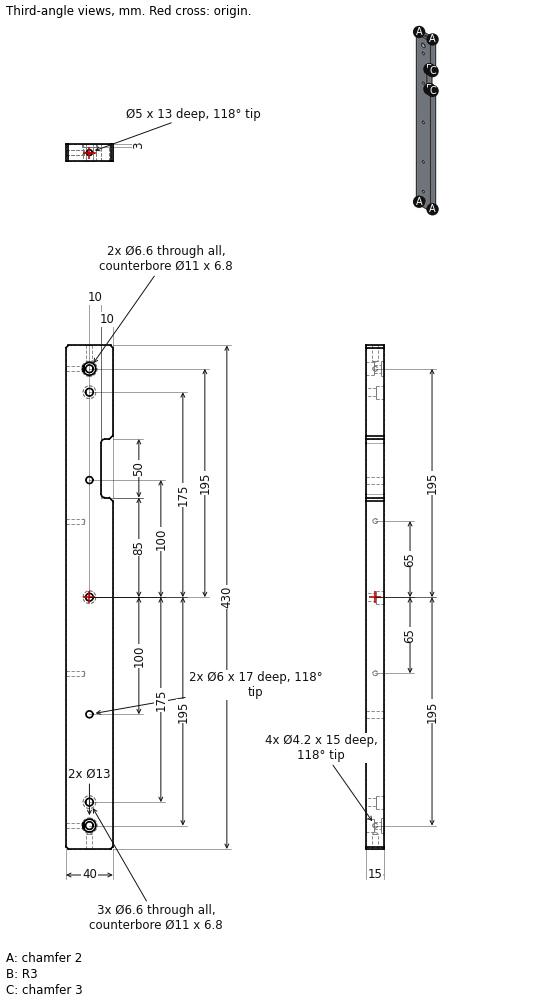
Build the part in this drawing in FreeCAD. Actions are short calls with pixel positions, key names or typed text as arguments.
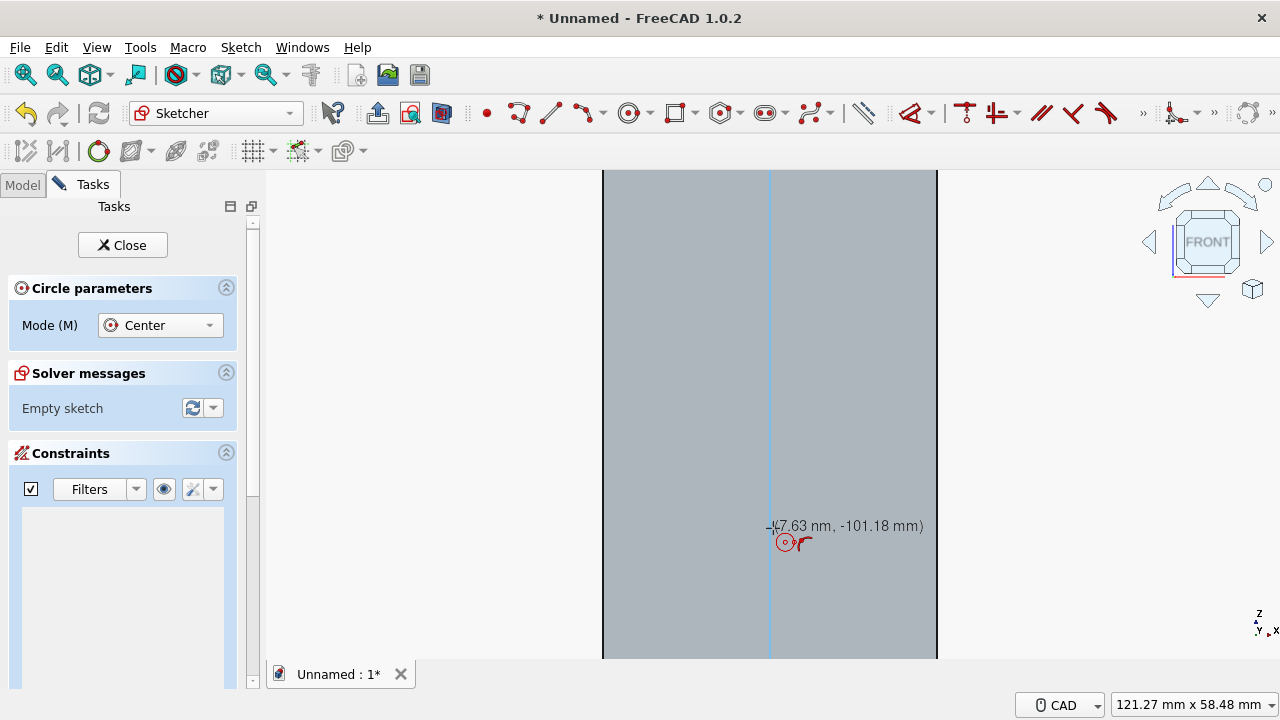
scroll(692, 559, down, 9)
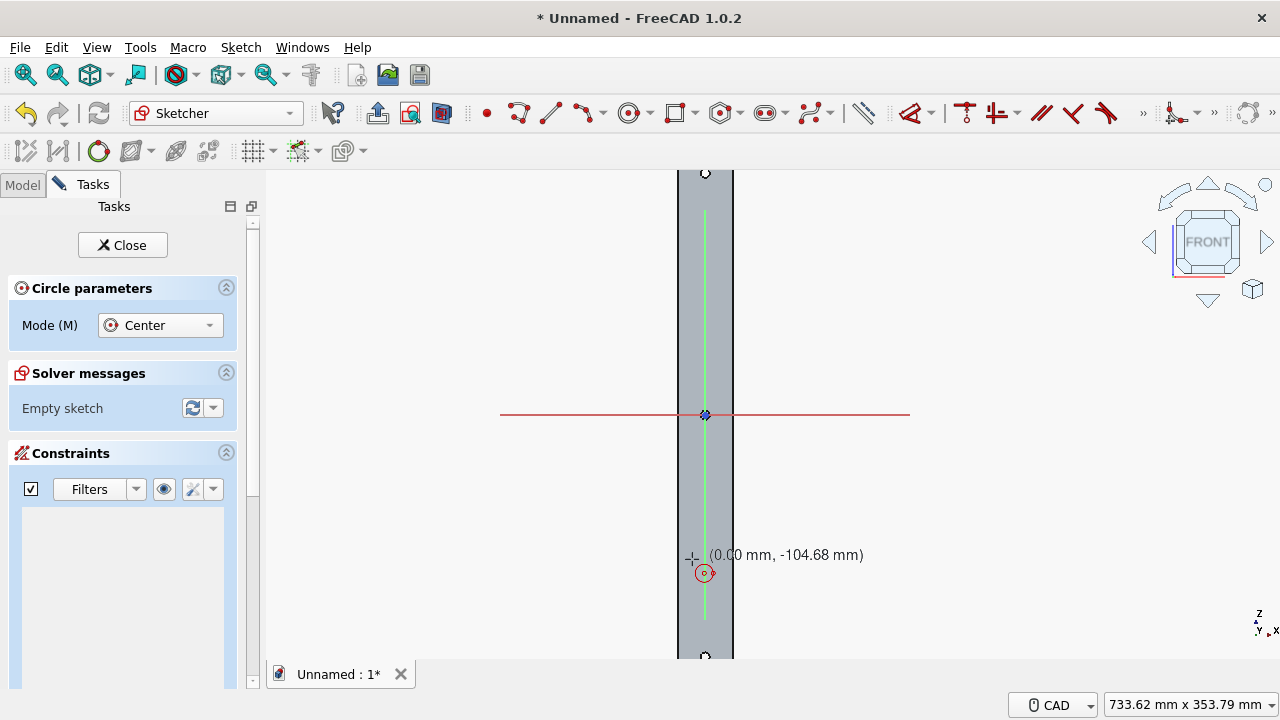
click(705, 553)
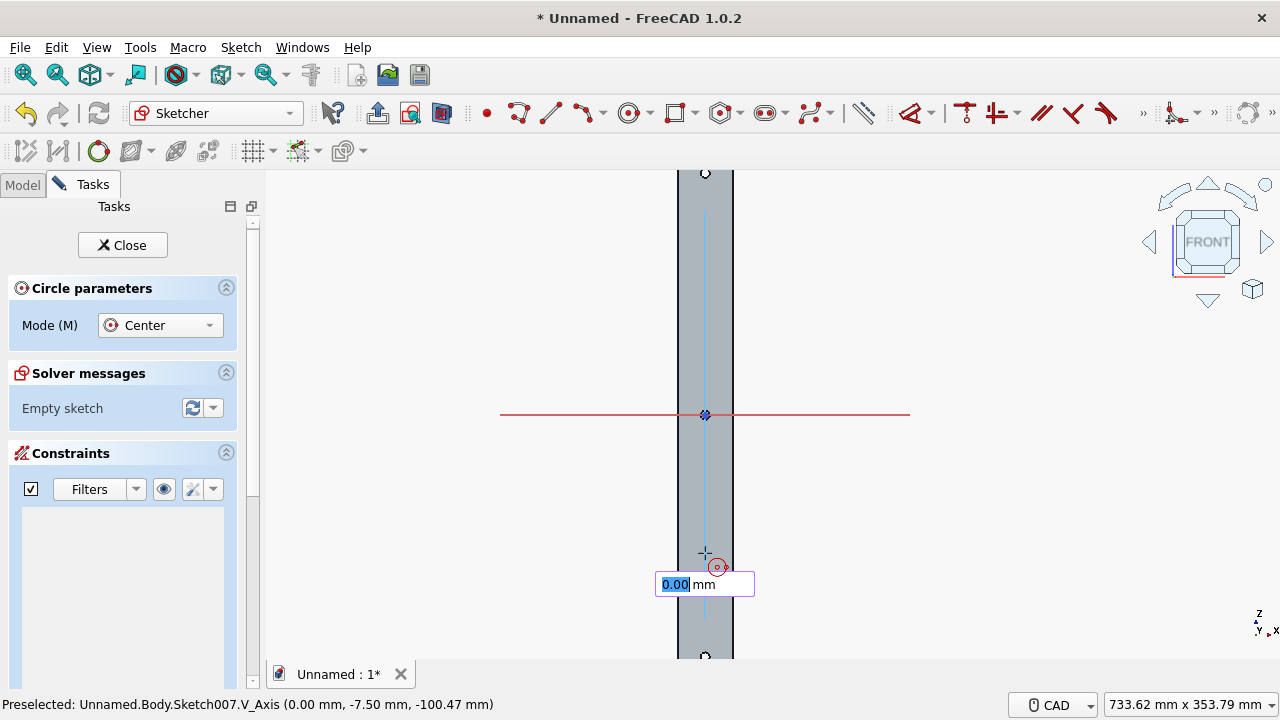
scroll(709, 552, up, 8)
move(708, 549)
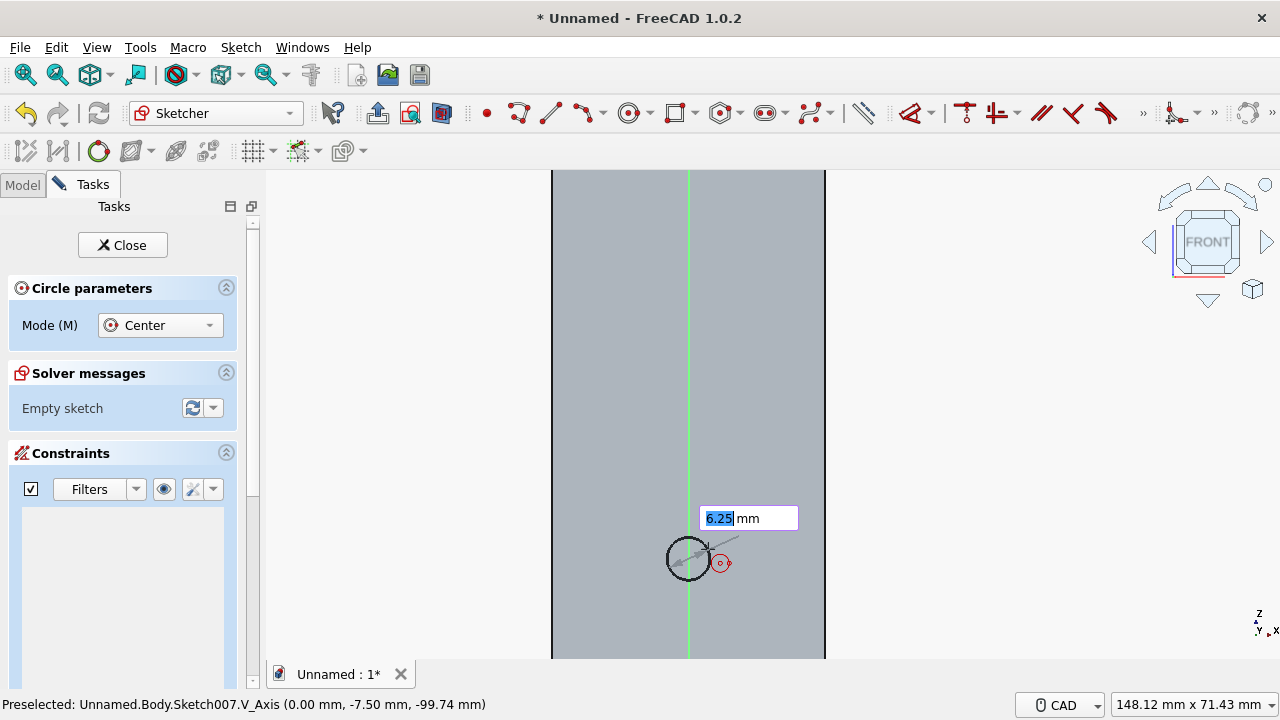
text(6)
key(Return)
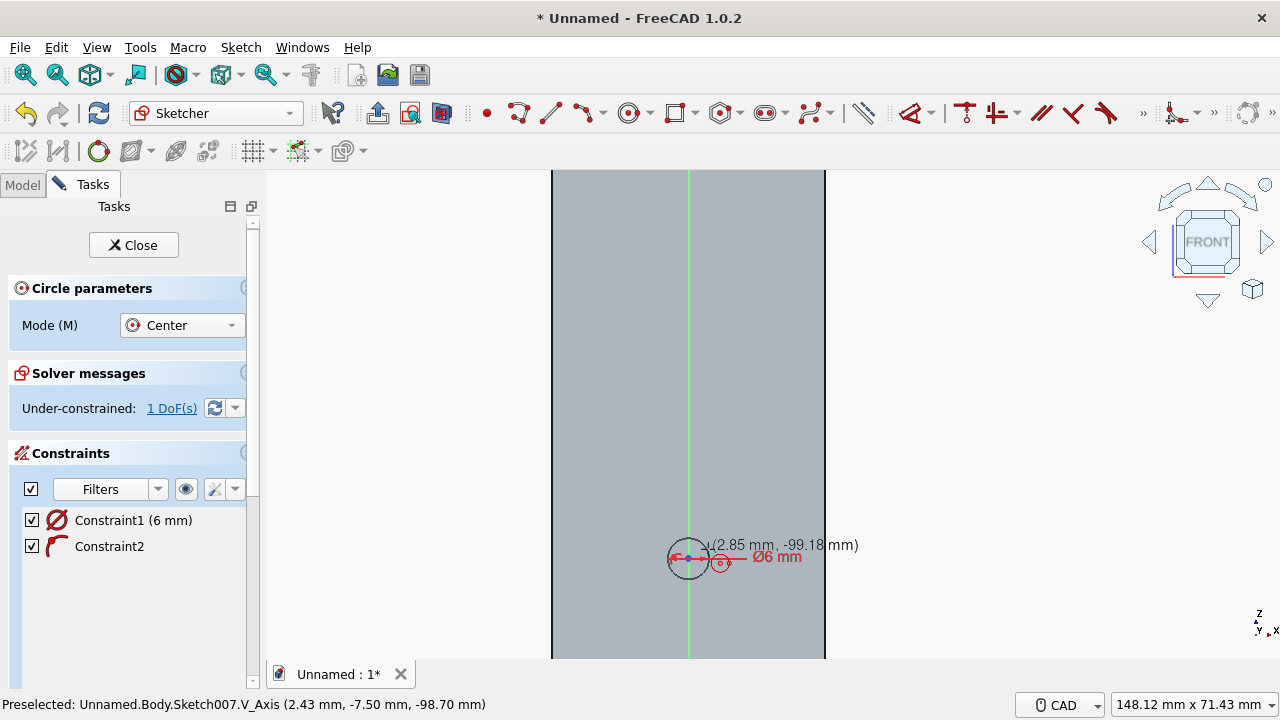
scroll(709, 552, down, 8)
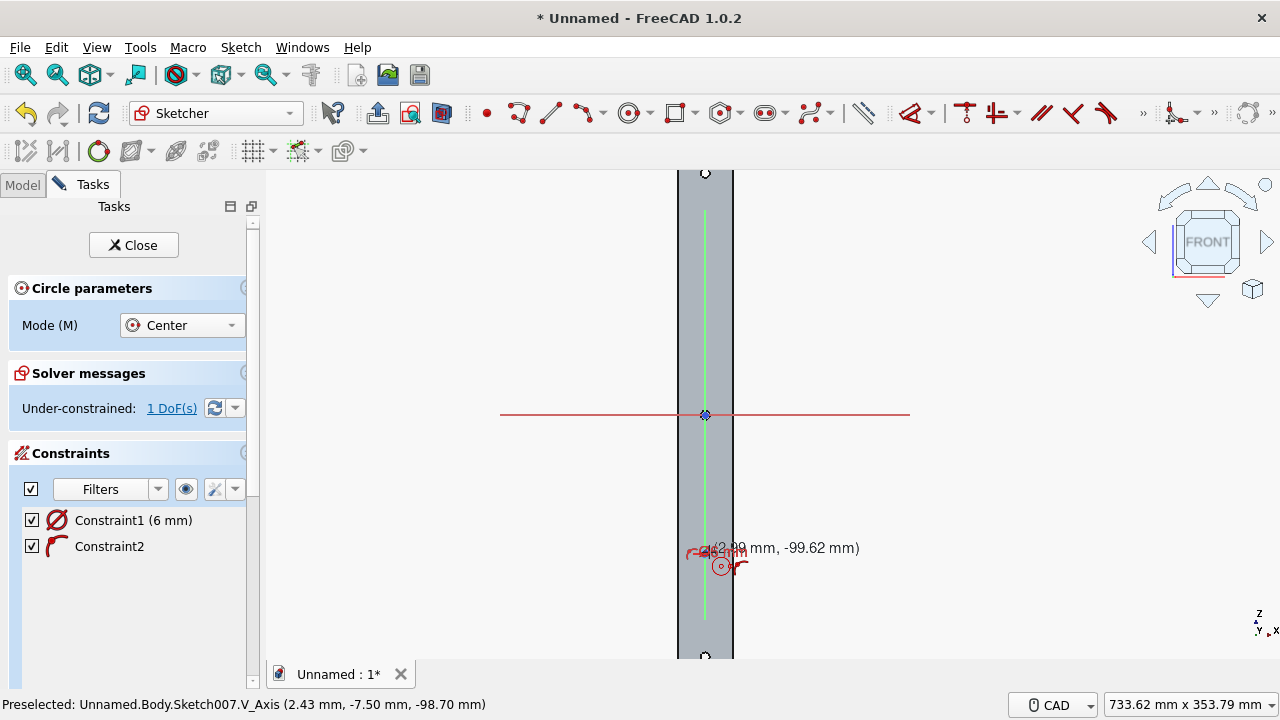
scroll(705, 277, up, 9)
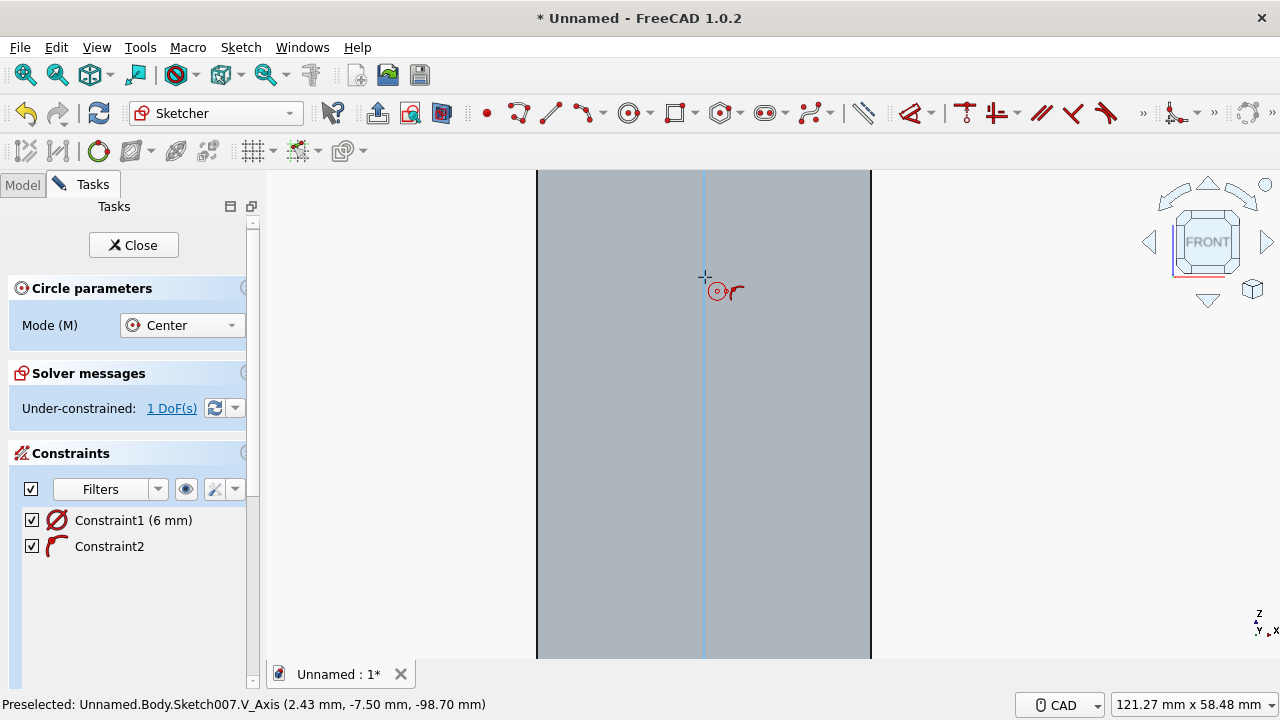
scroll(705, 276, down, 9)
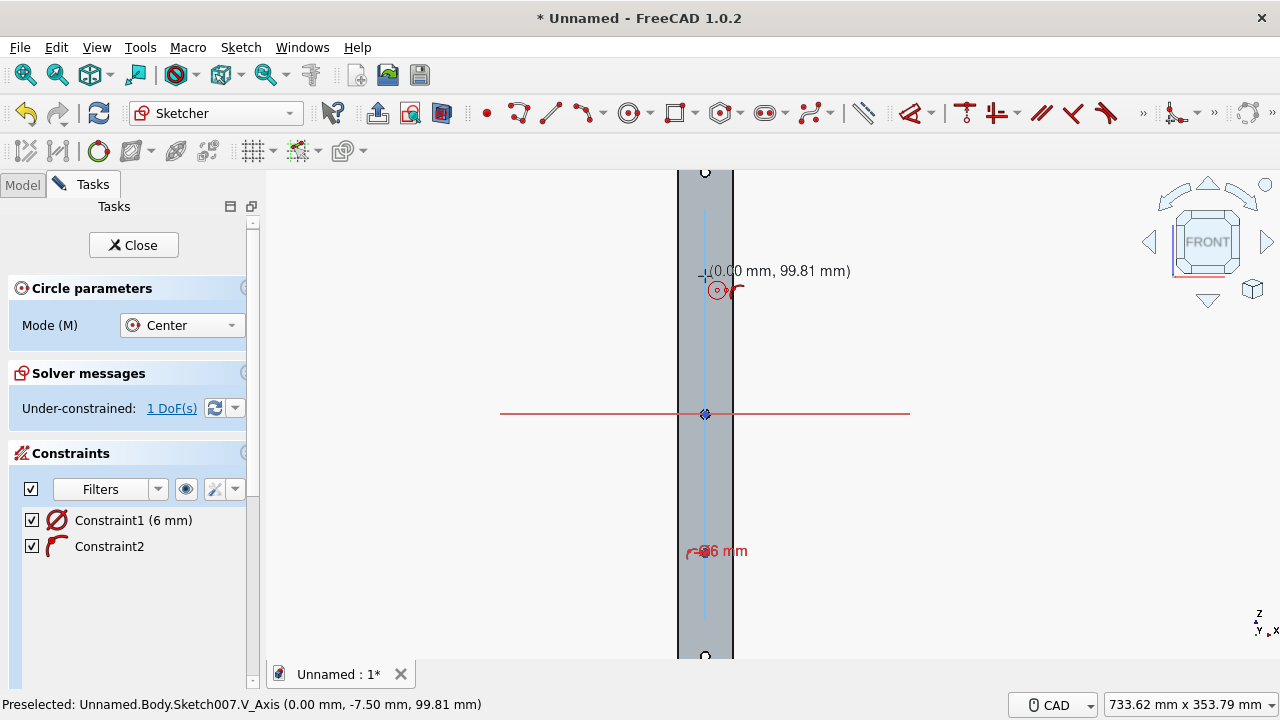
click(705, 276)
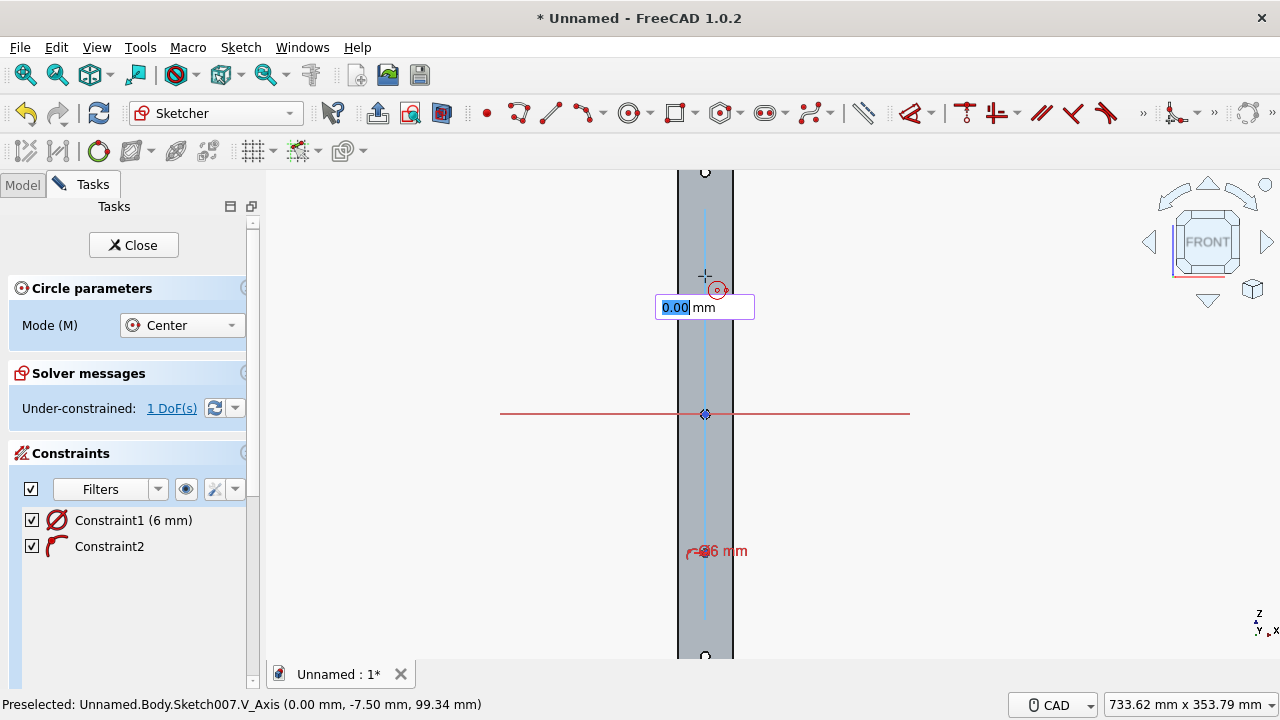
scroll(709, 275, up, 8)
move(708, 272)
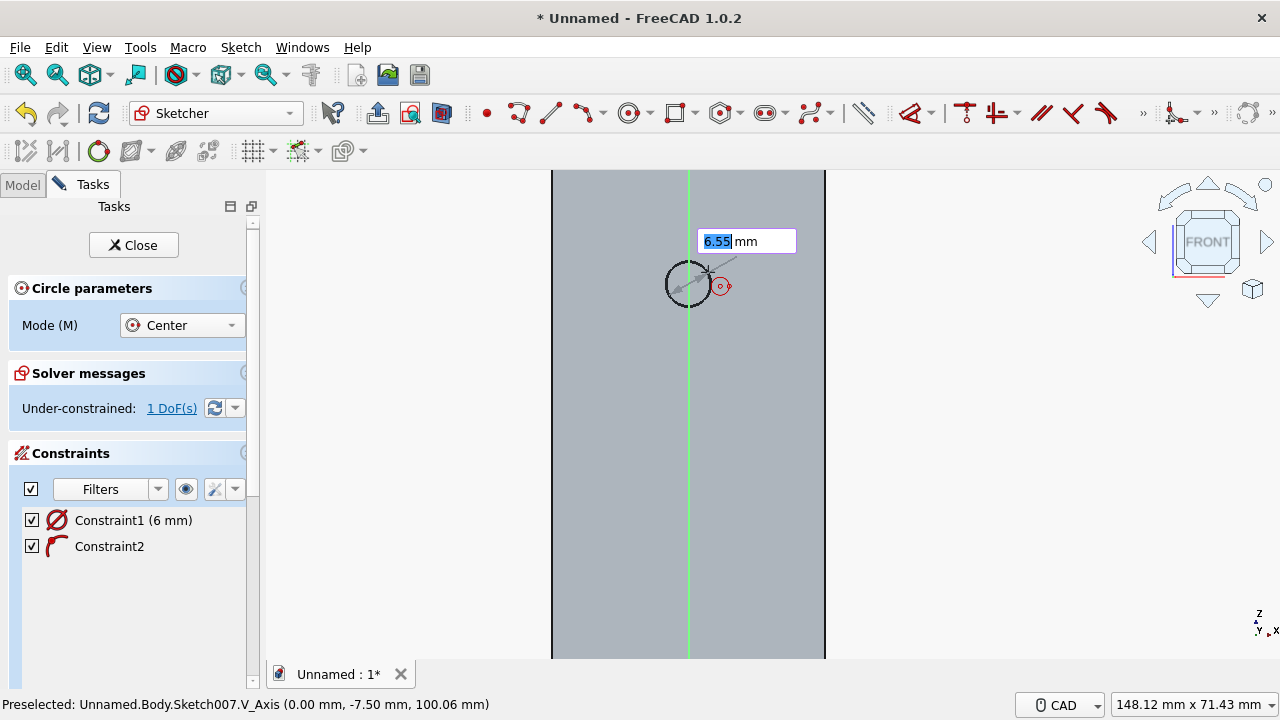
text(6)
key(Return)
key(Escape)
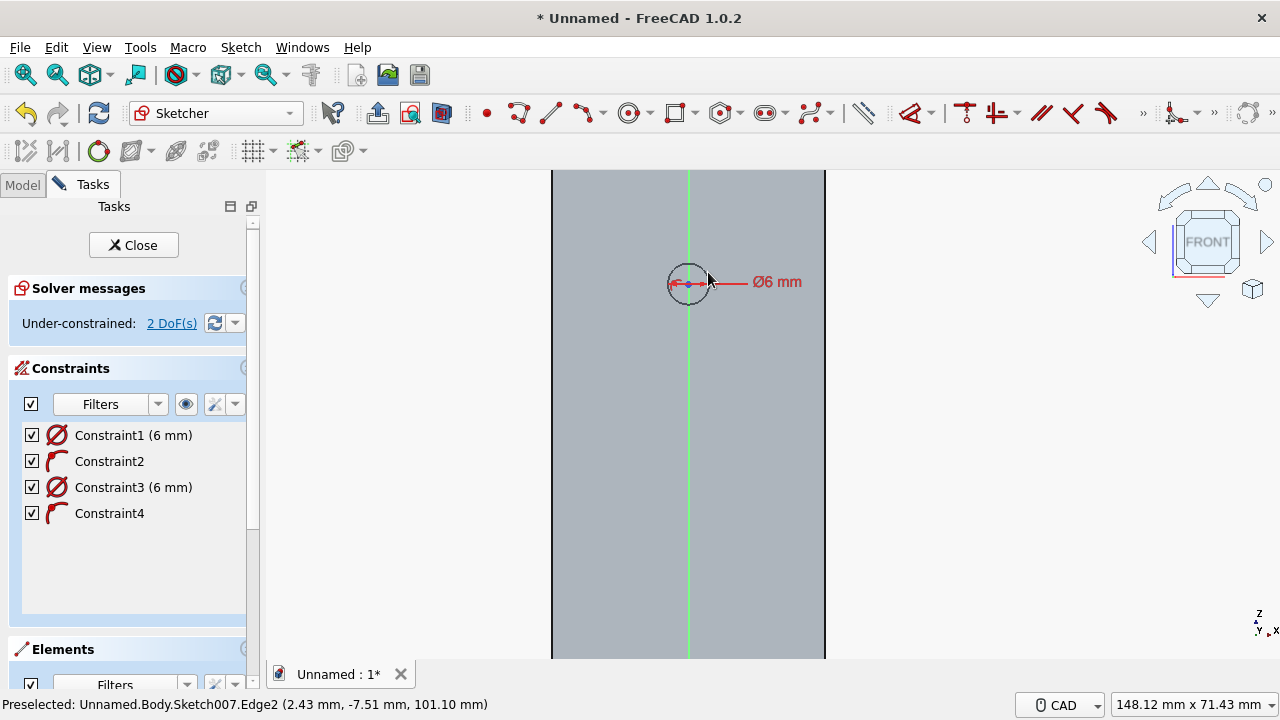
click(910, 114)